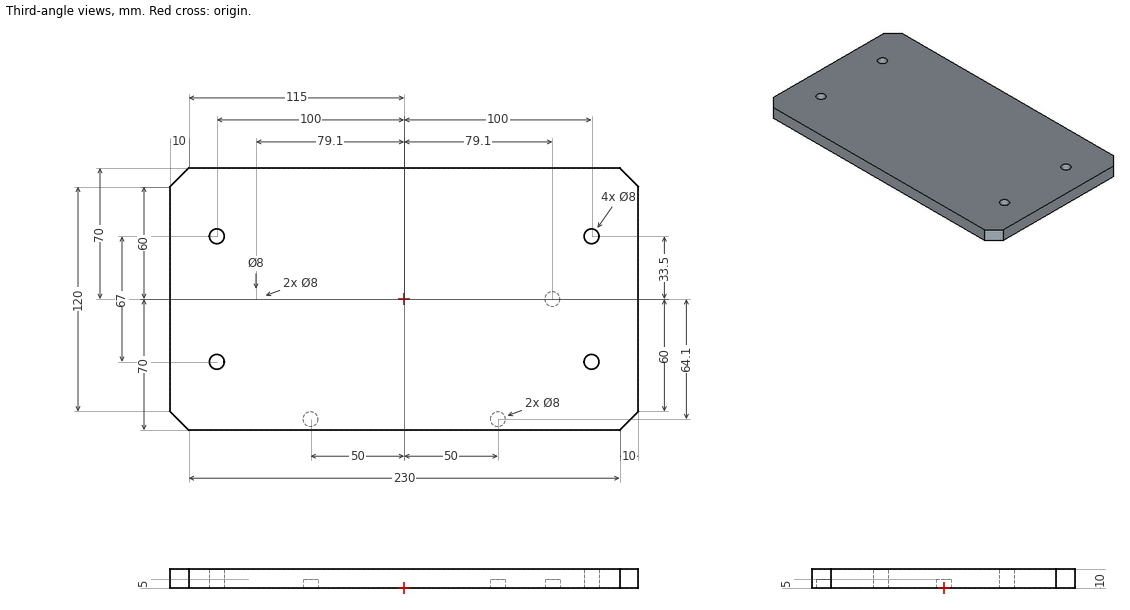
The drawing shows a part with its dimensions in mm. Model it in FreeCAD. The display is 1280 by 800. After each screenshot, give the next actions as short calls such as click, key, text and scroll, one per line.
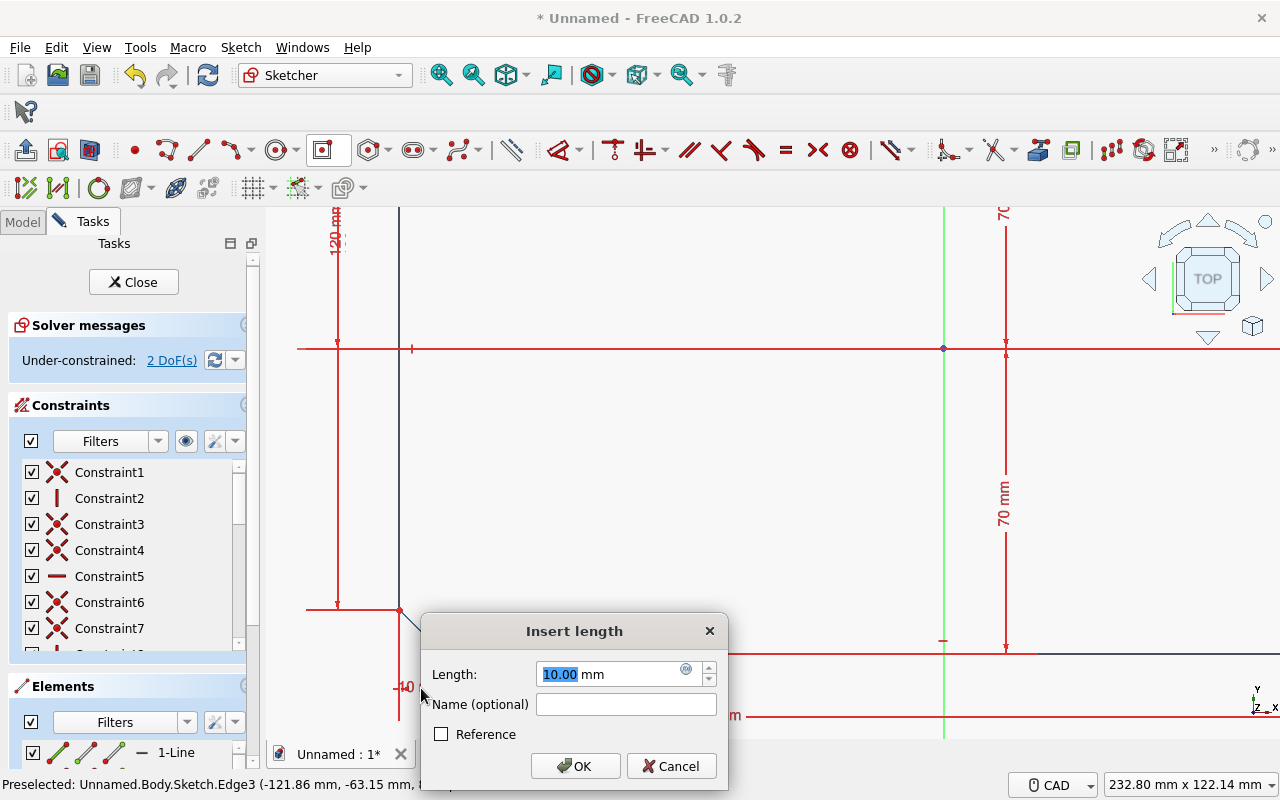
text(10)
key(Return)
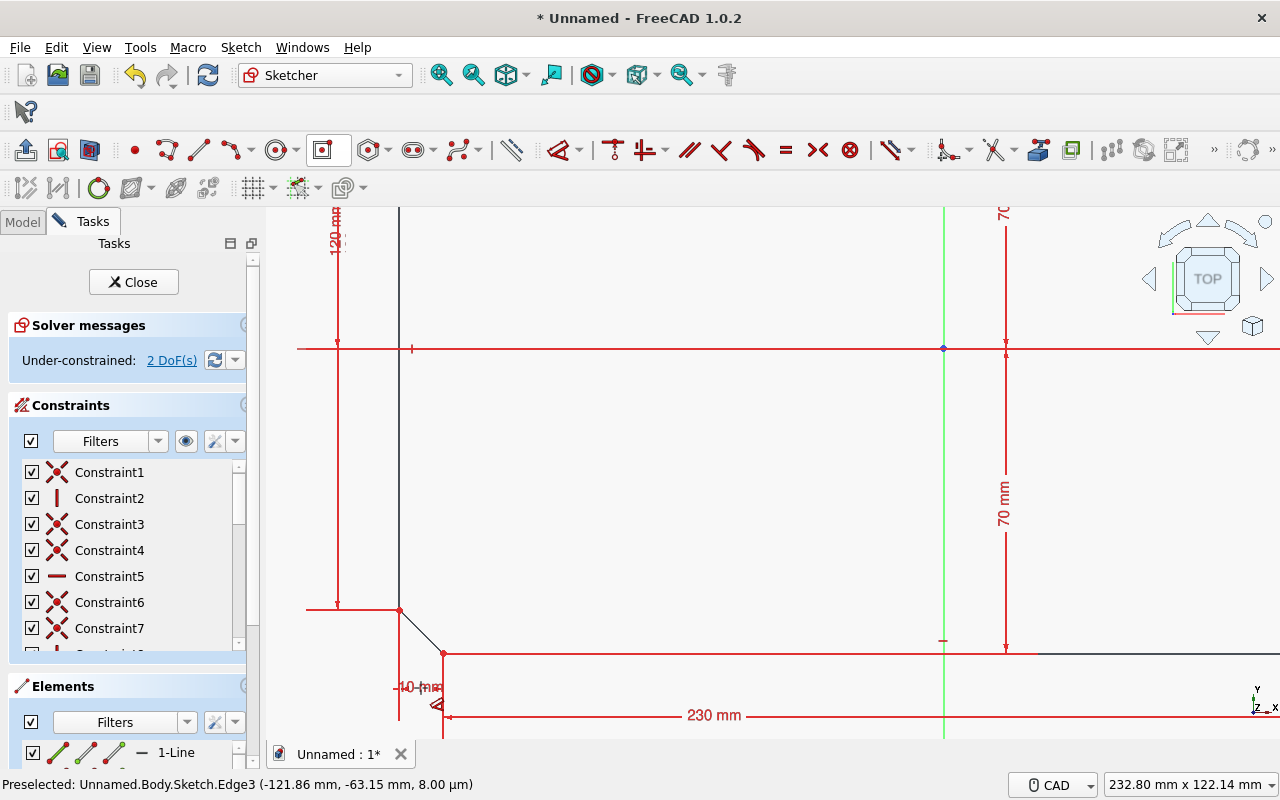
scroll(413, 624, down, 3)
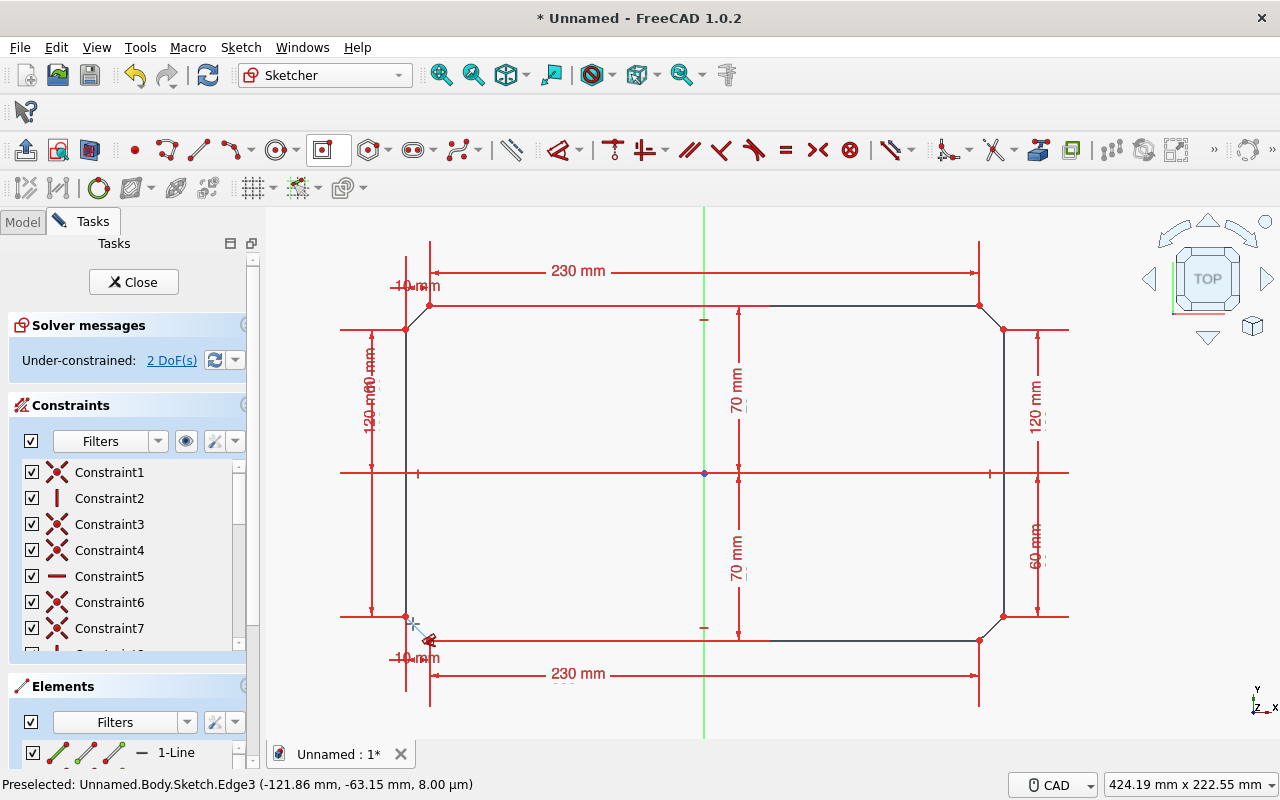
scroll(987, 633, up, 3)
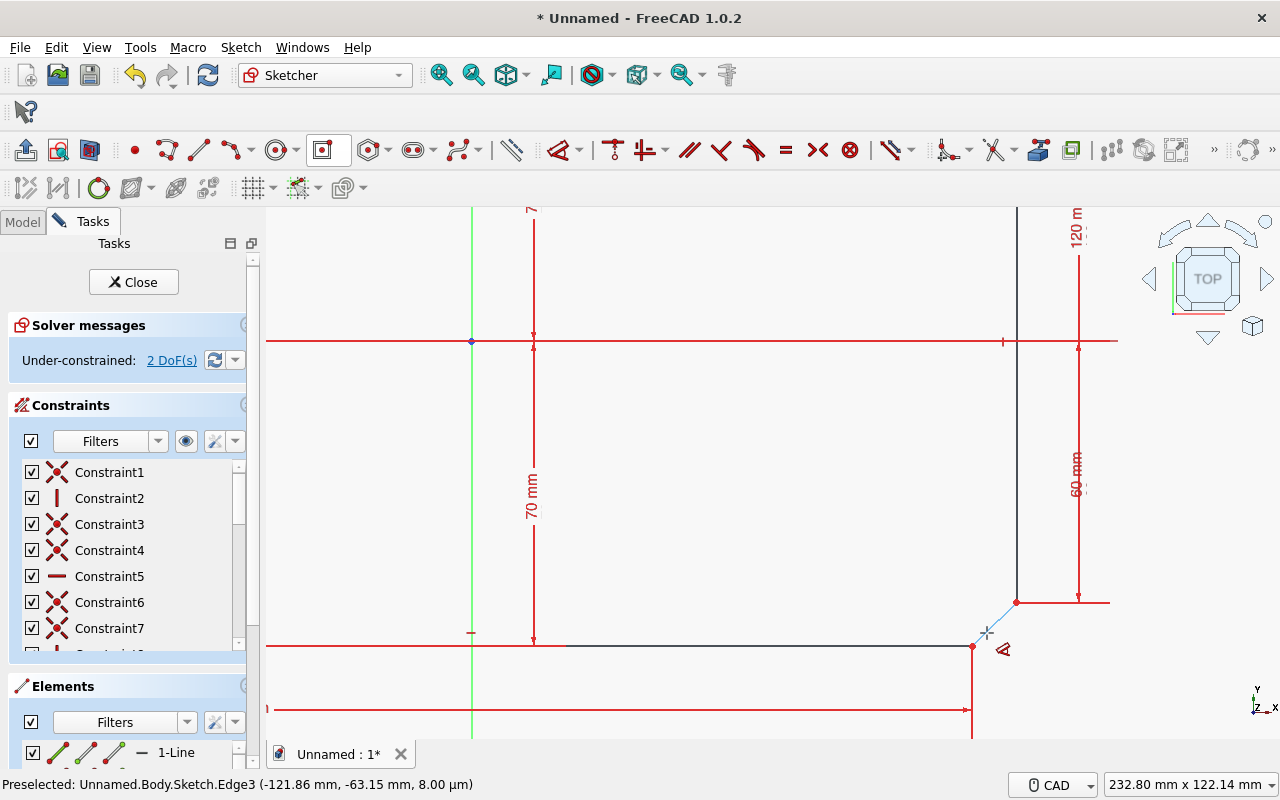
click(986, 633)
click(995, 680)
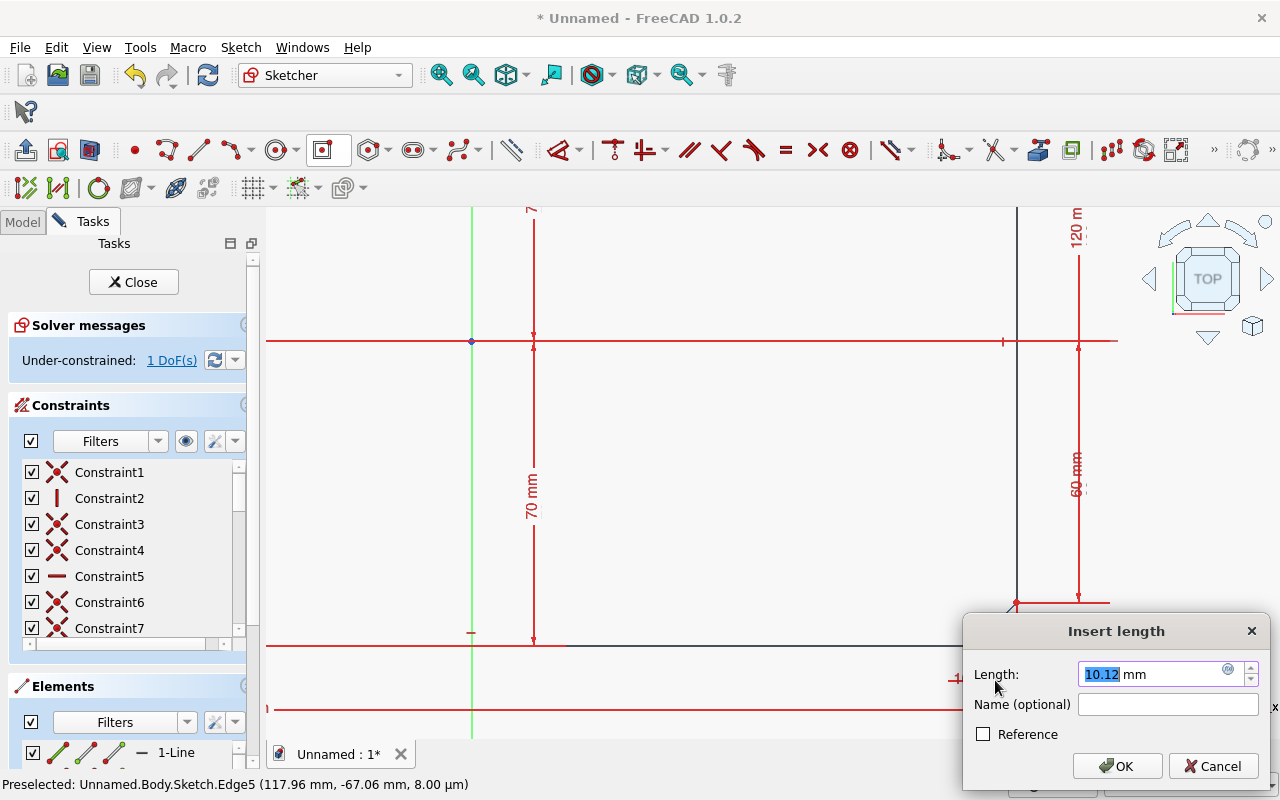
text(10)
key(Return)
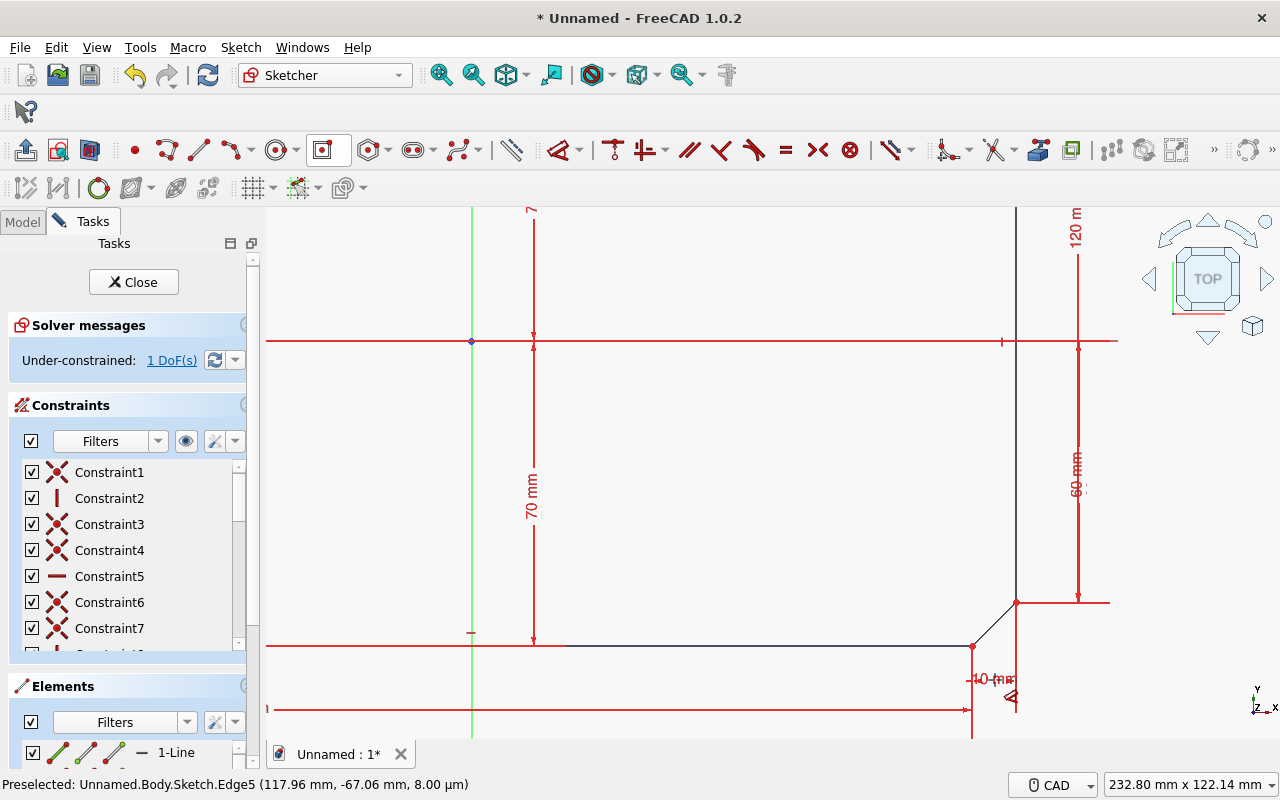
scroll(988, 633, down, 3)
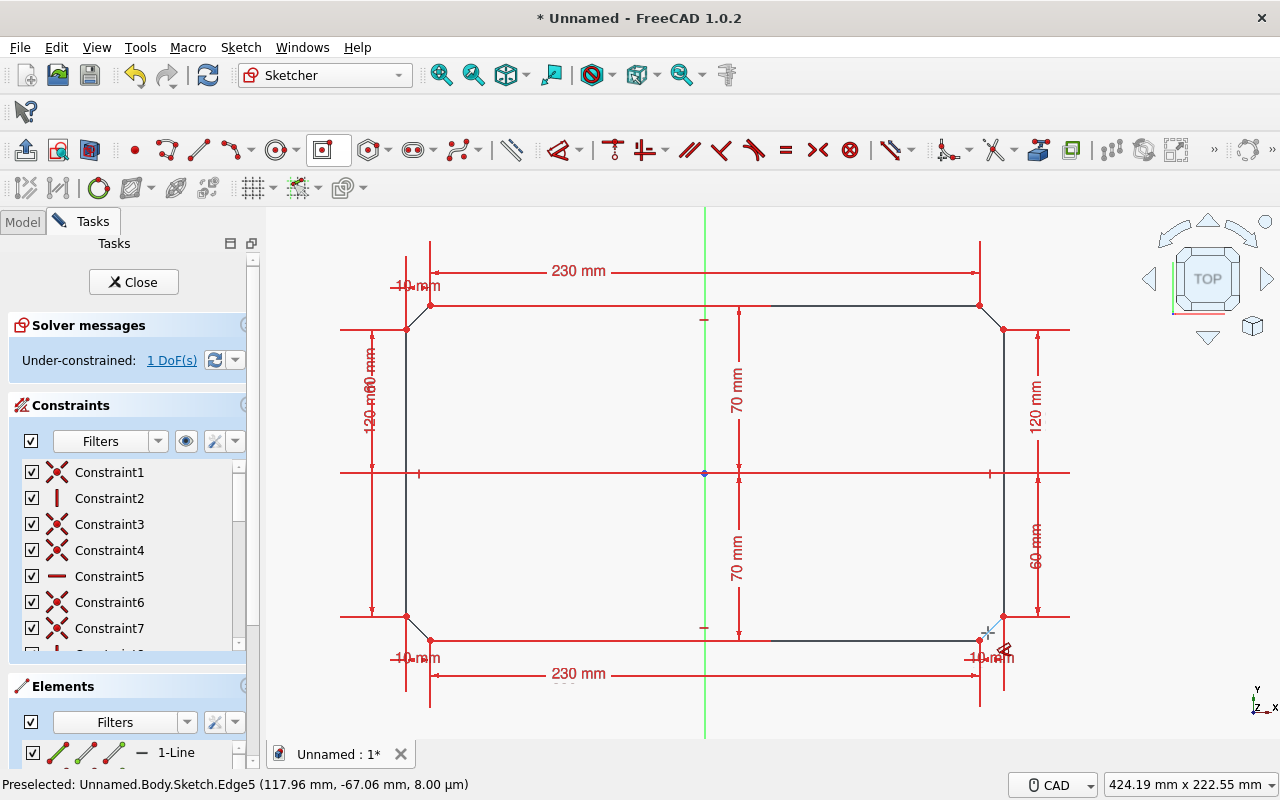
click(430, 306)
click(504, 272)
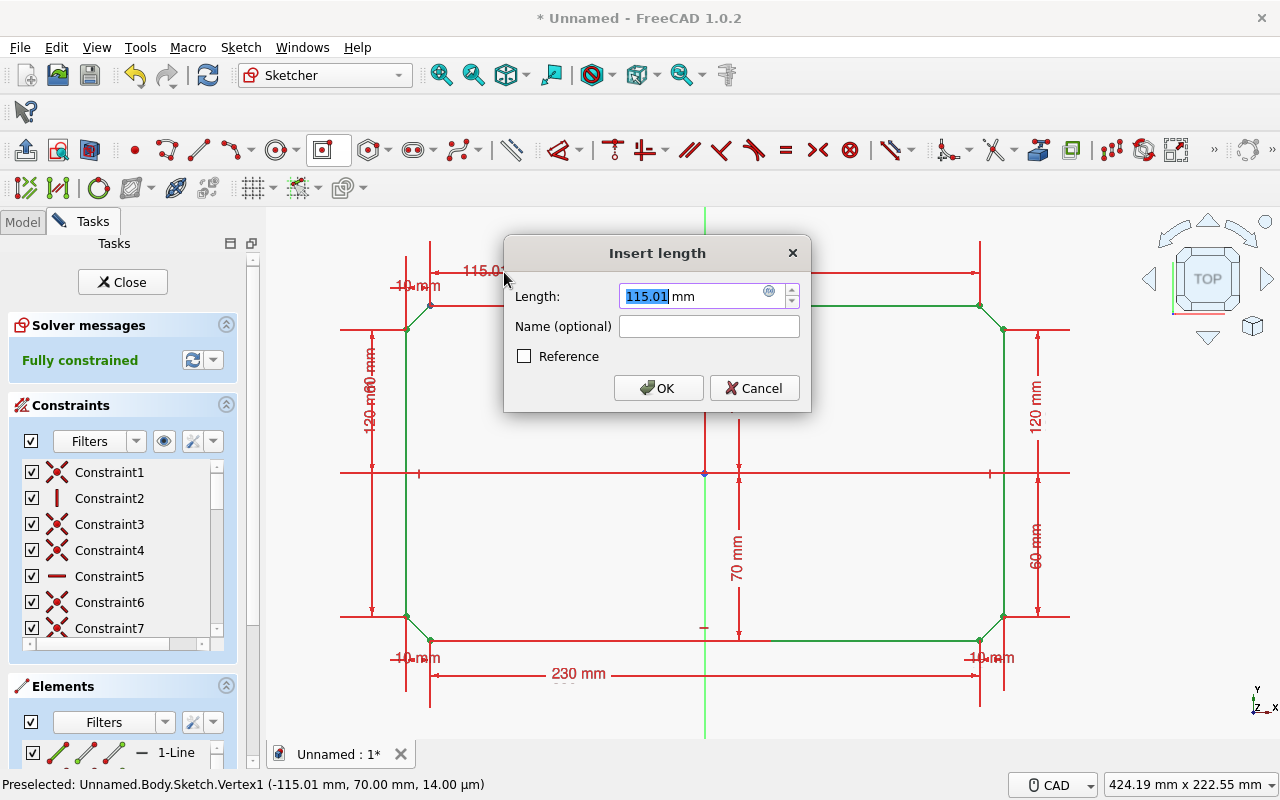
text(115)
key(Return)
key(Escape)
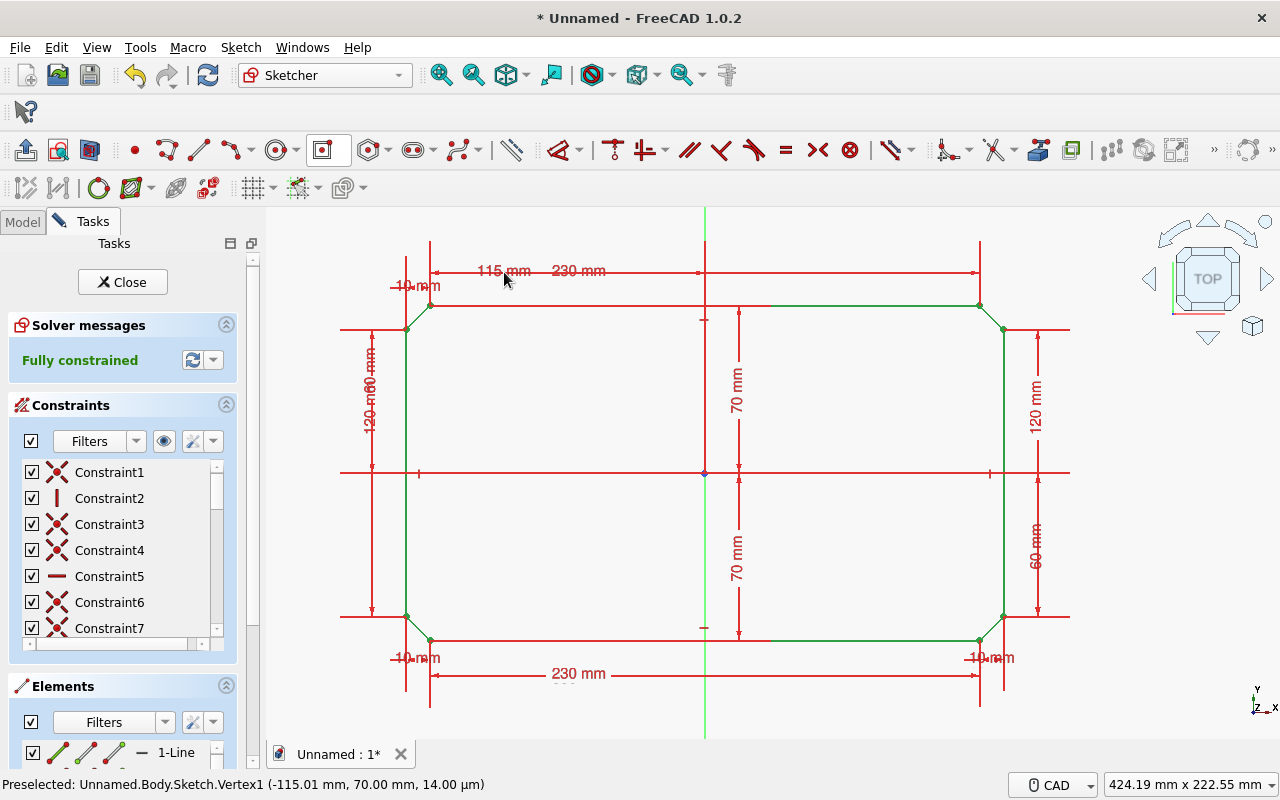
click(123, 282)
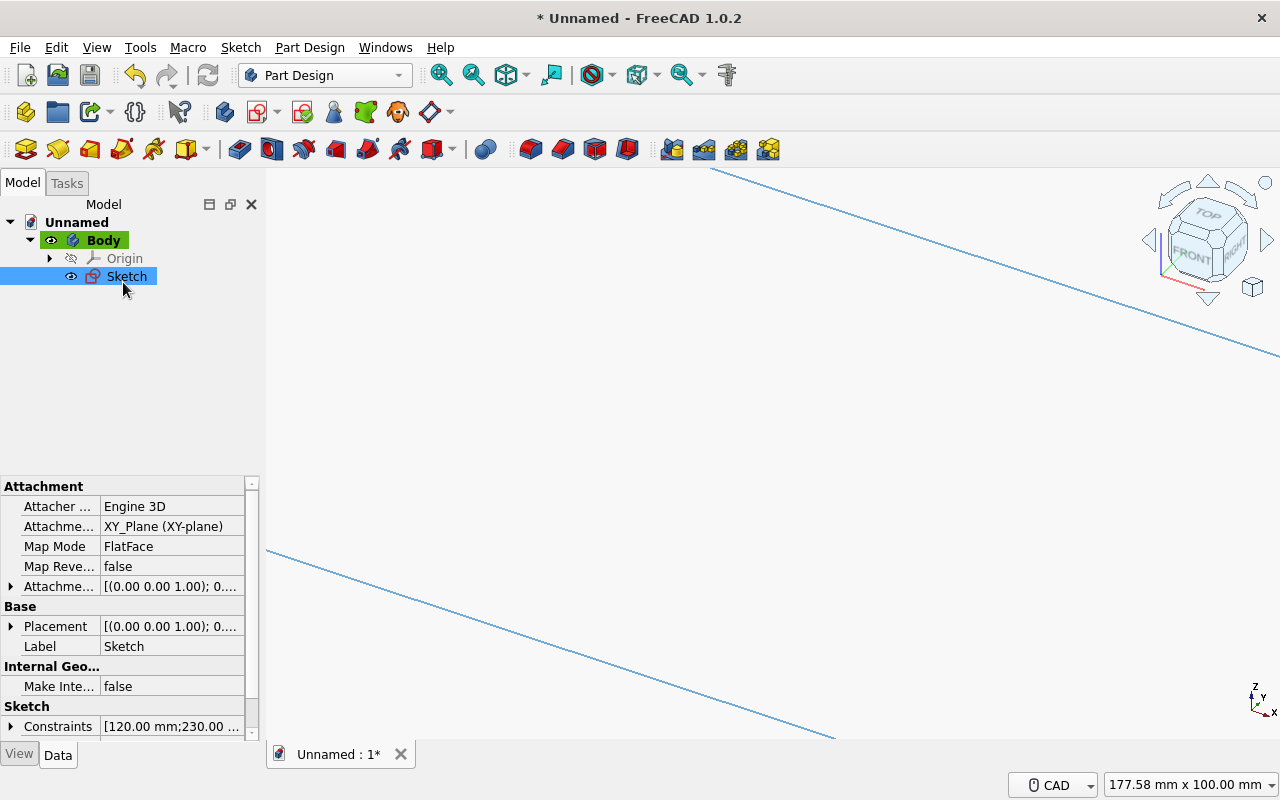
click(26, 150)